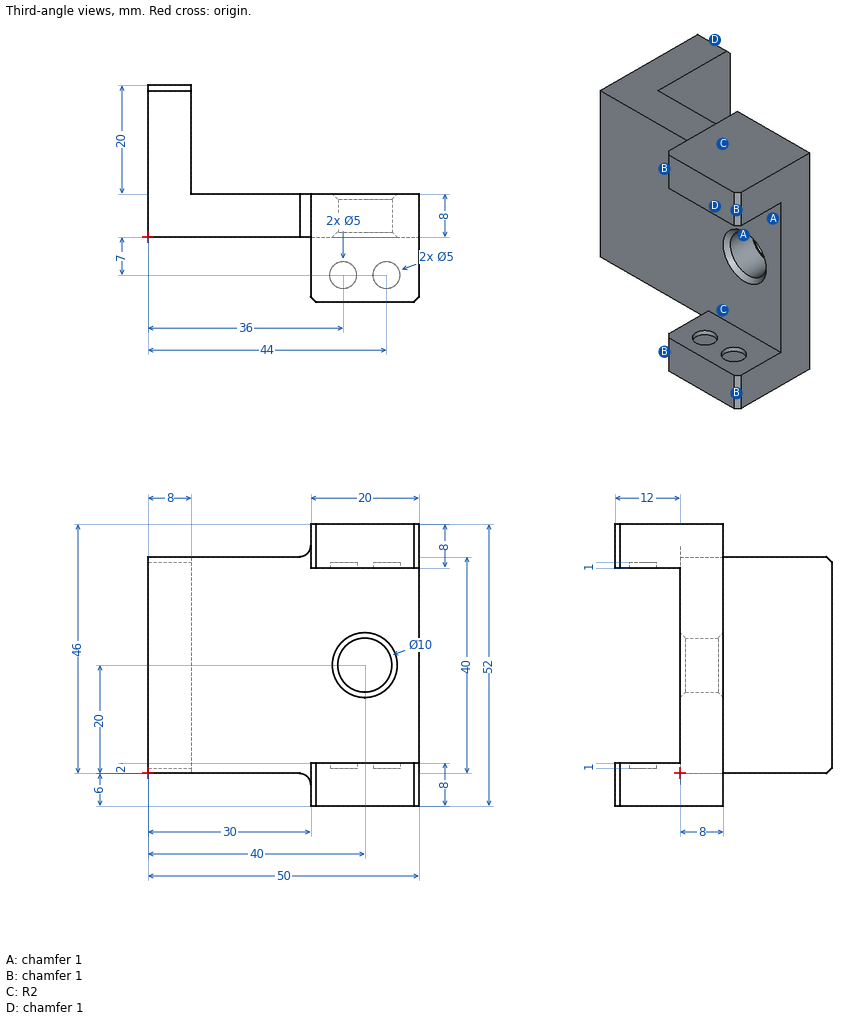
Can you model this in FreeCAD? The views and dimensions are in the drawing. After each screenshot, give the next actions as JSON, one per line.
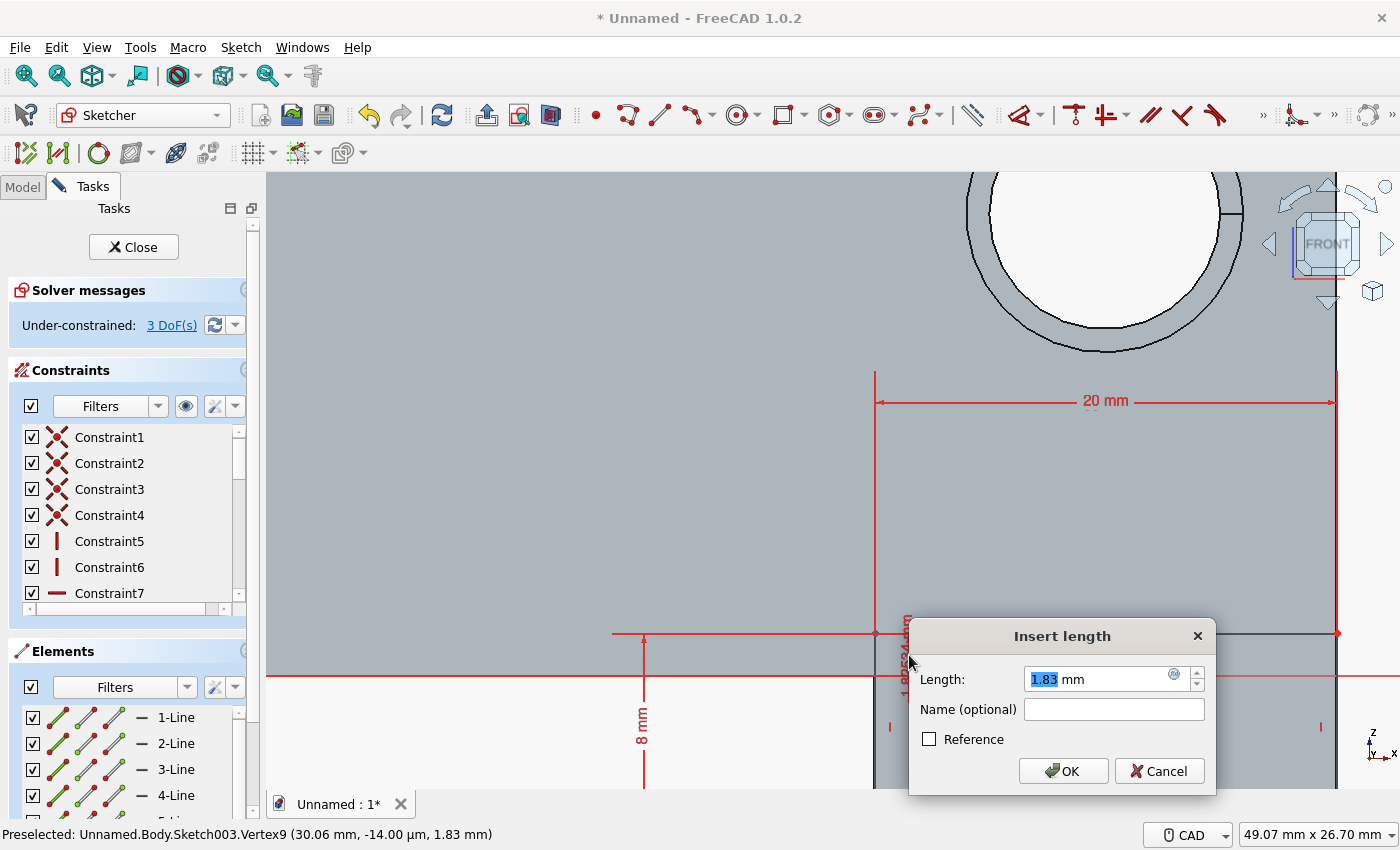
{"action": "type", "text": "2"}
{"action": "key", "text": "Return"}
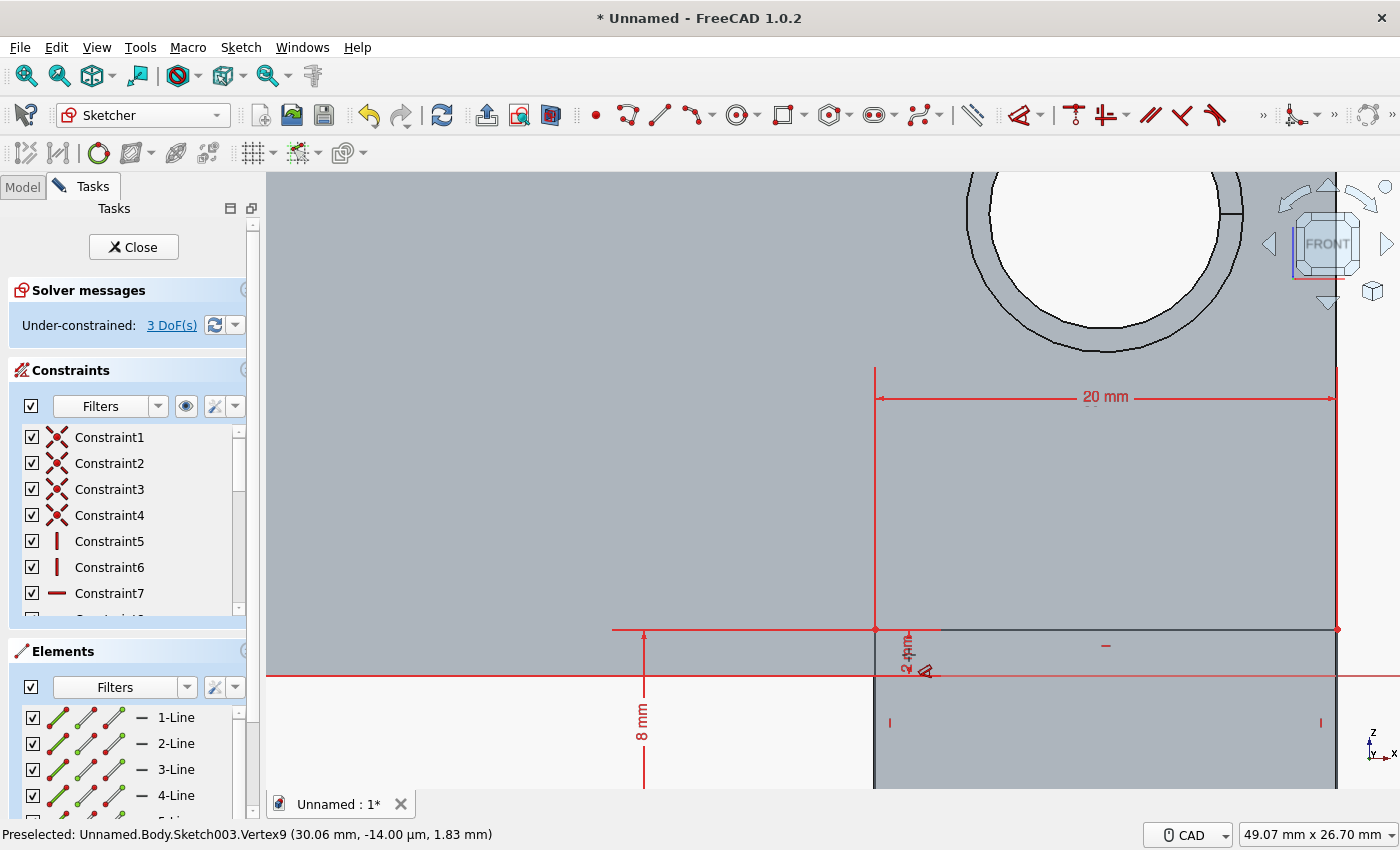
{"action": "scroll", "coordinate": [767, 595], "scroll_direction": "down", "scroll_amount": 6}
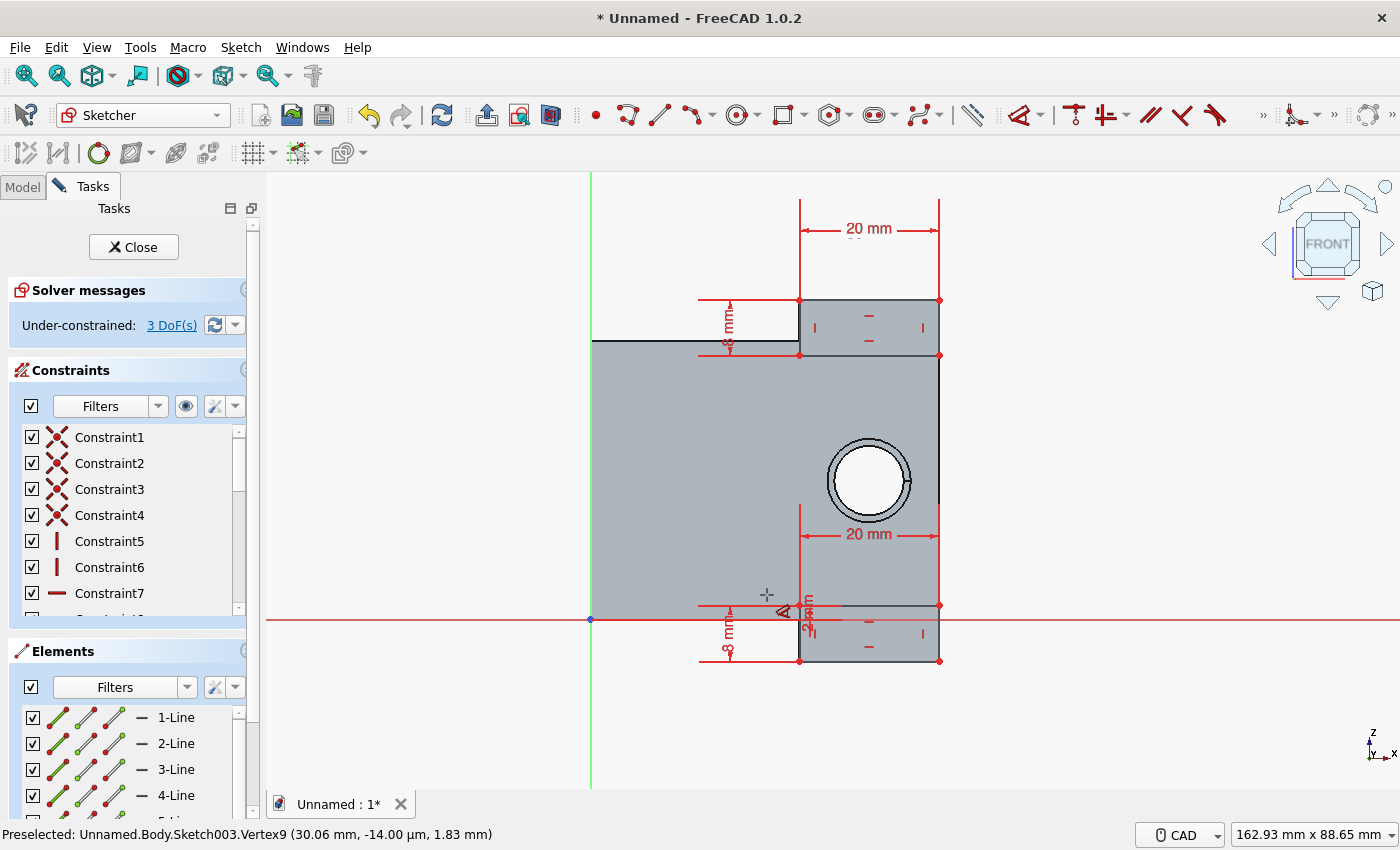
{"action": "left_click", "coordinate": [800, 300]}
{"action": "left_click", "coordinate": [695, 266]}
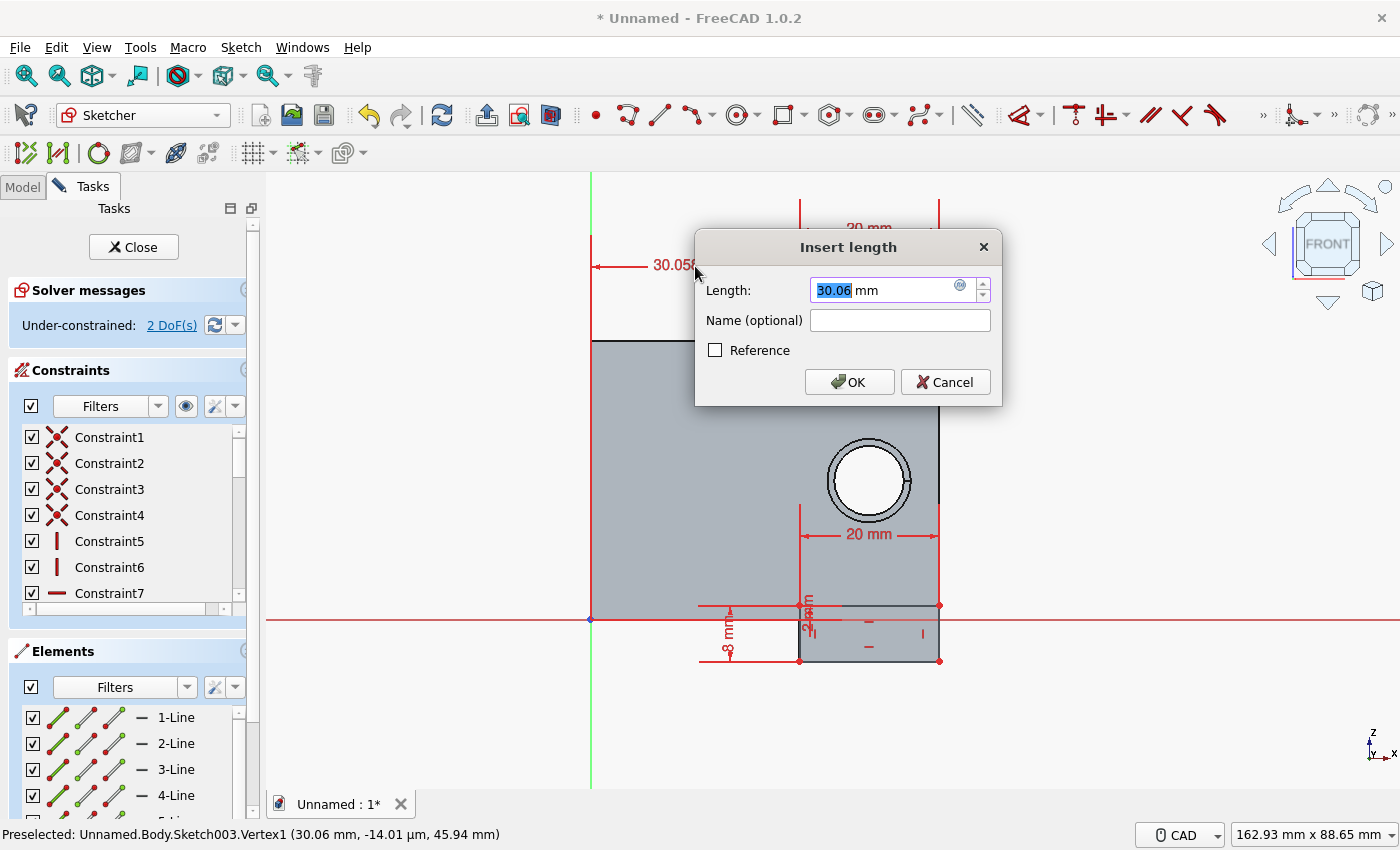
{"action": "type", "text": "30"}
{"action": "key", "text": "Return"}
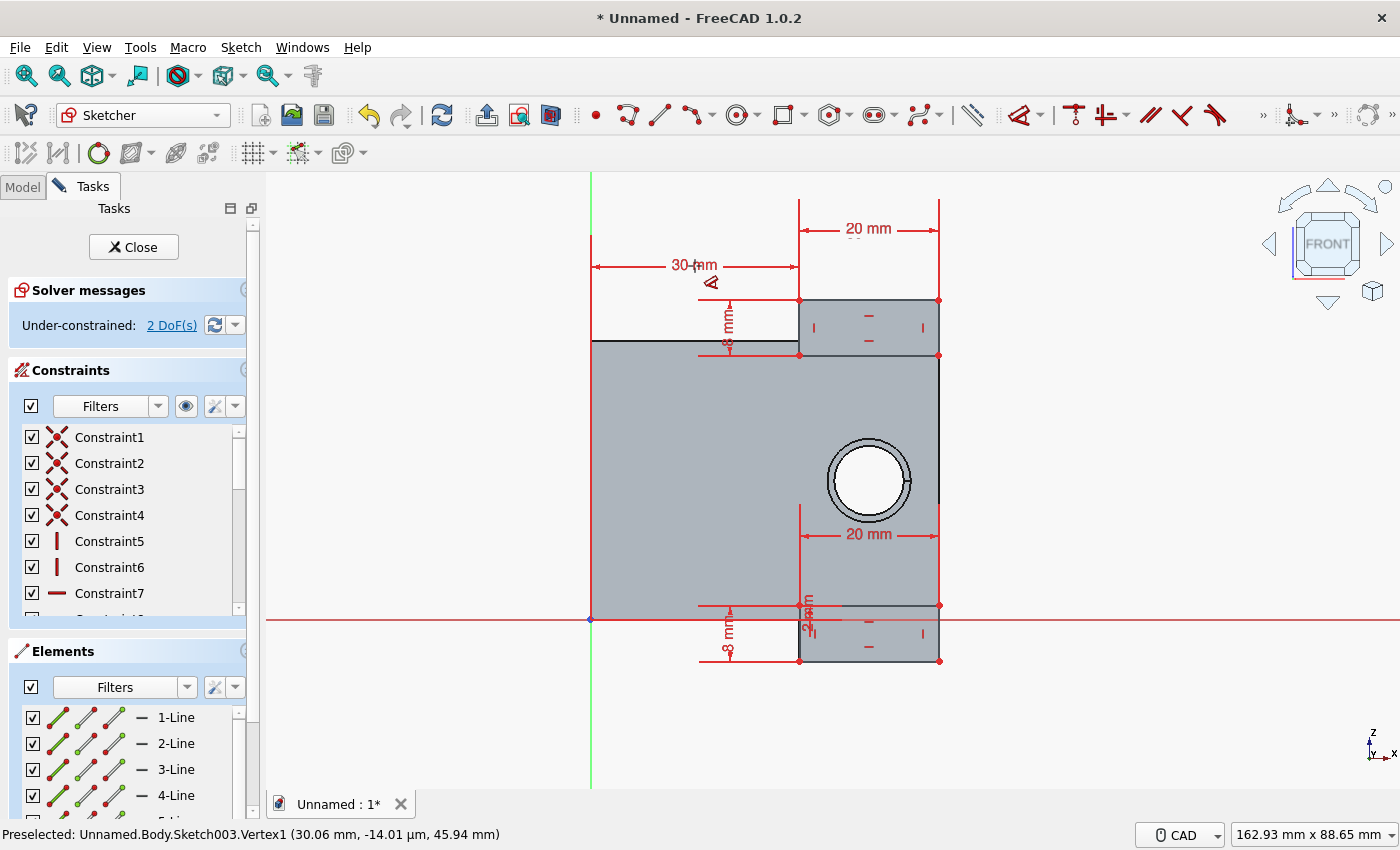
{"action": "left_click", "coordinate": [799, 300]}
{"action": "left_click", "coordinate": [557, 460]}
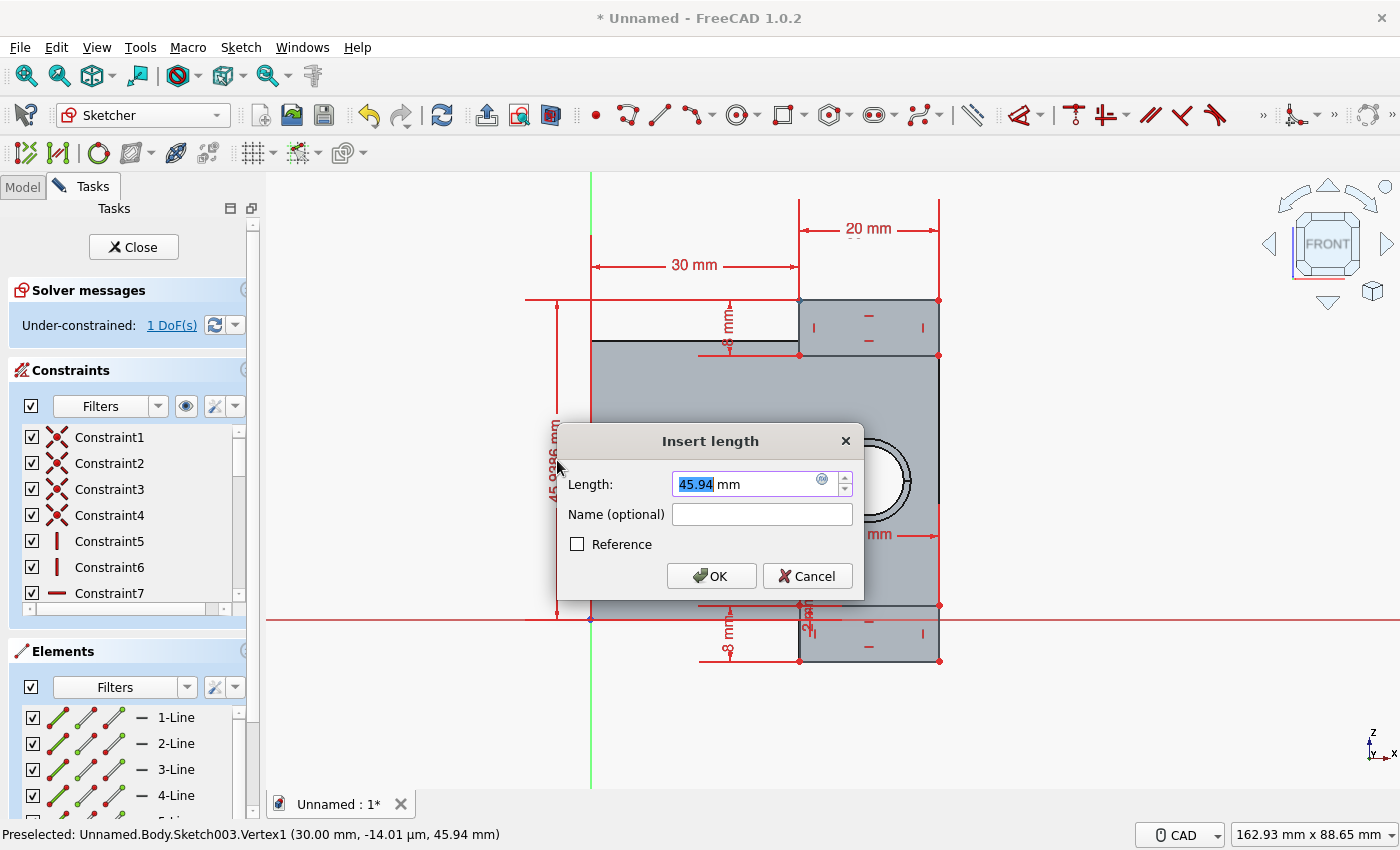
{"action": "type", "text": "46"}
{"action": "key", "text": "Return"}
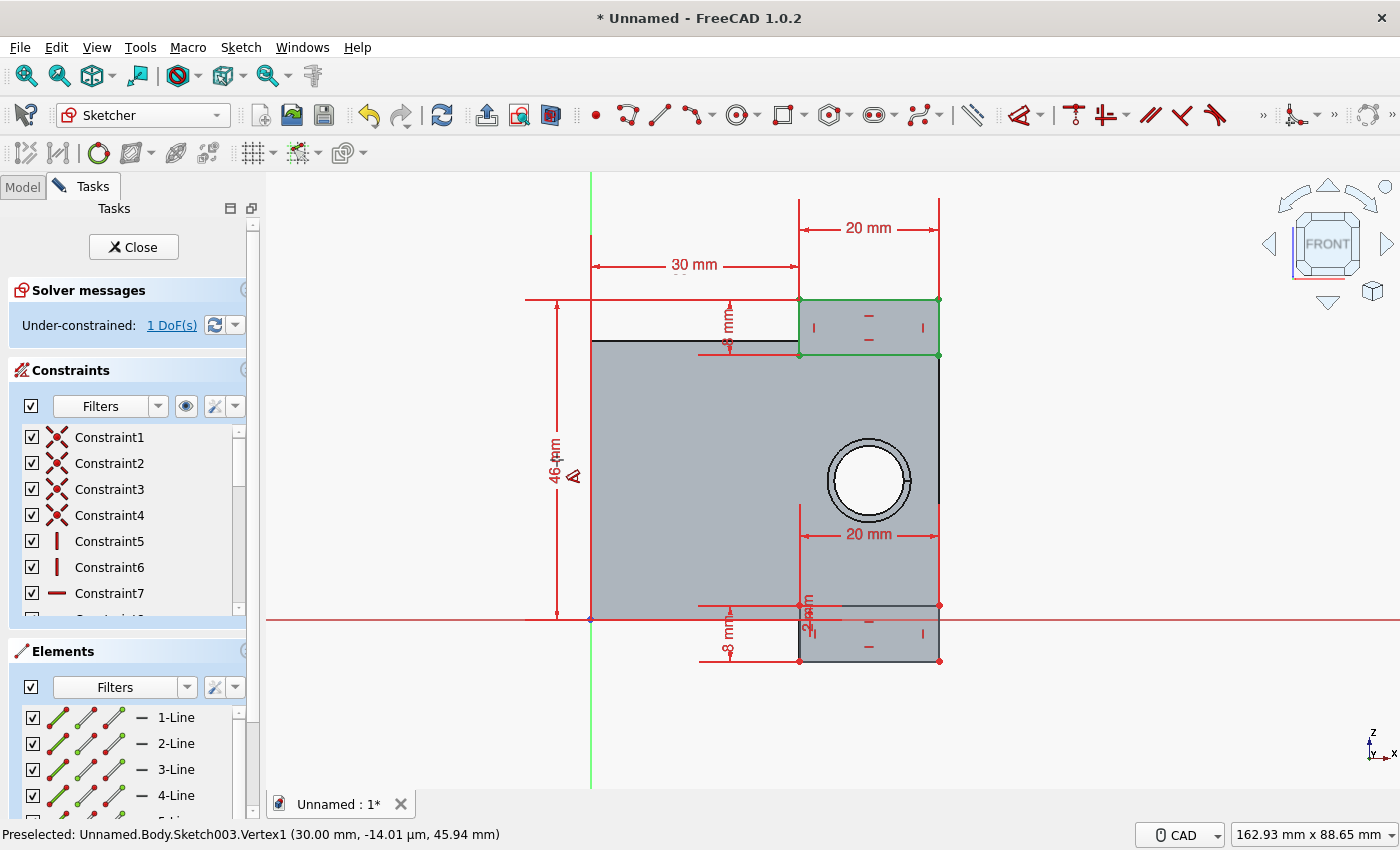
{"action": "left_click", "coordinate": [800, 606]}
{"action": "left_click", "coordinate": [695, 654]}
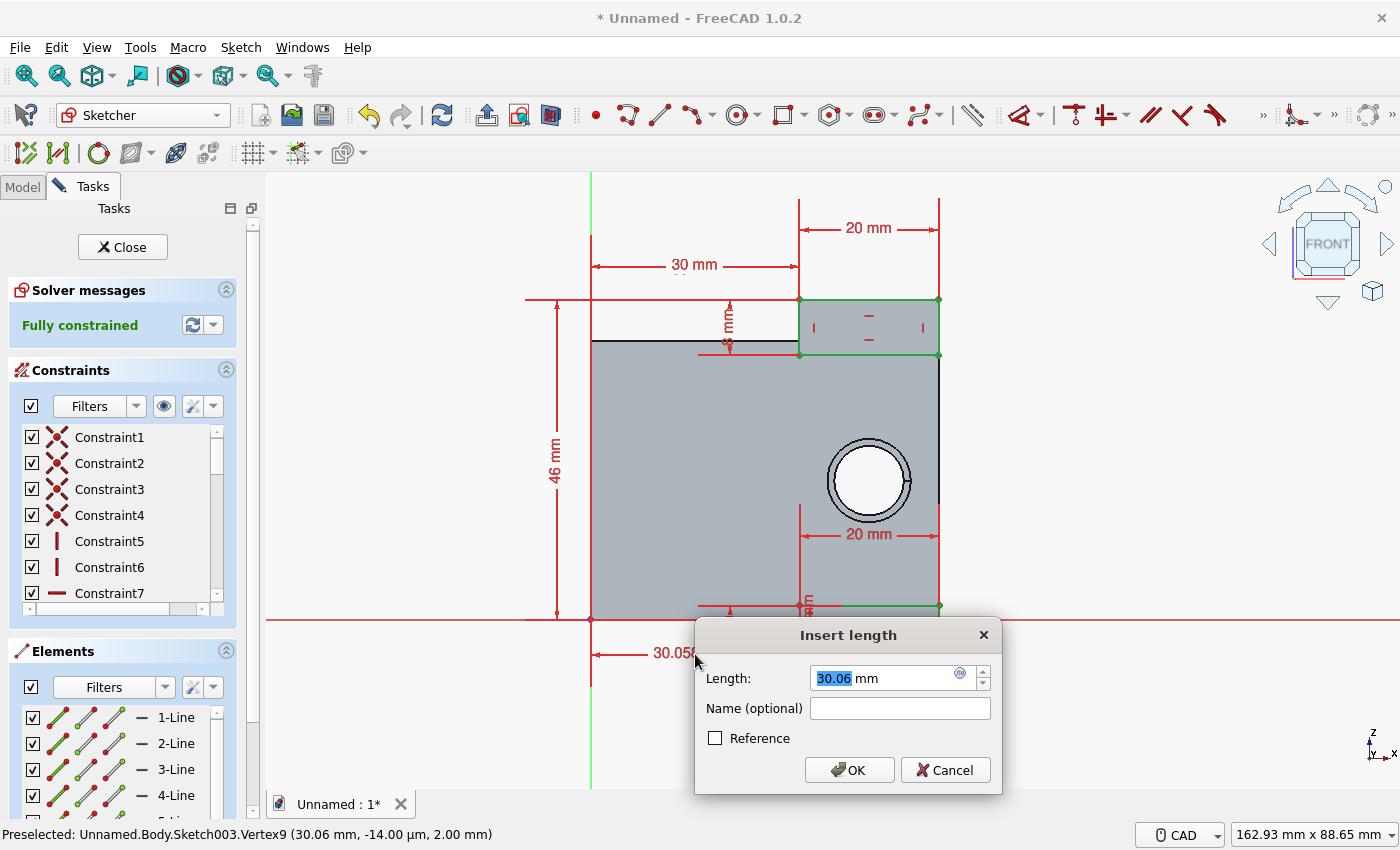
{"action": "type", "text": "30"}
{"action": "key", "text": "Return"}
{"action": "key", "text": "Escape"}